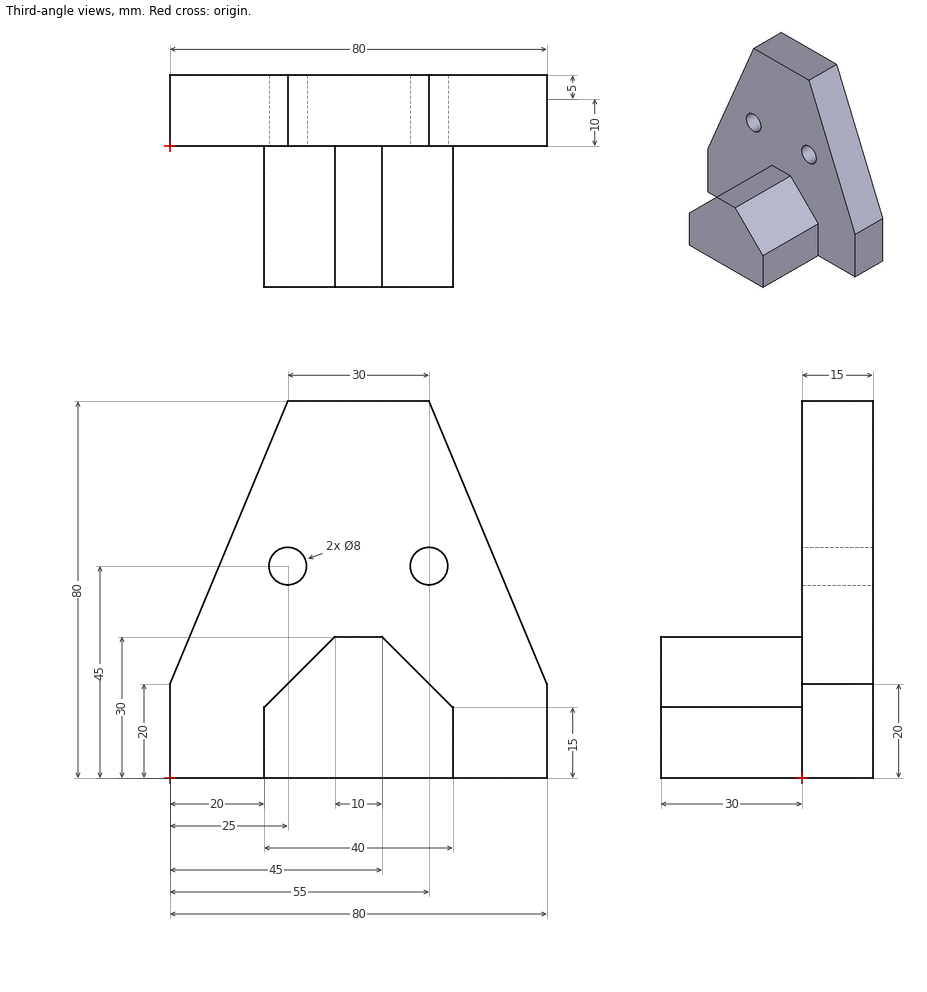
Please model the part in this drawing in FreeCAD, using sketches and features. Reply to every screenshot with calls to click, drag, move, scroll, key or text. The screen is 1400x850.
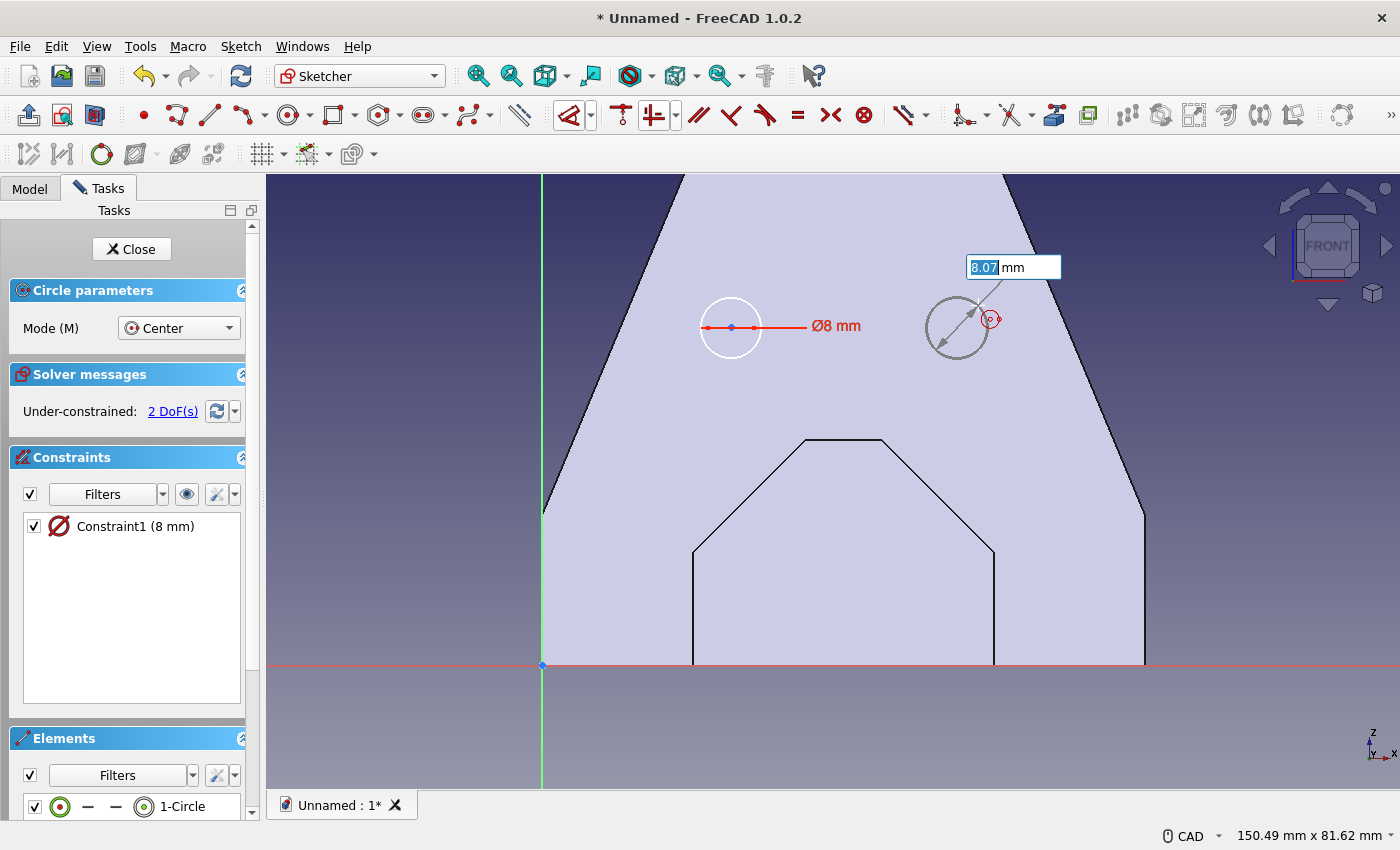
text(8)
key(Return)
key(Escape)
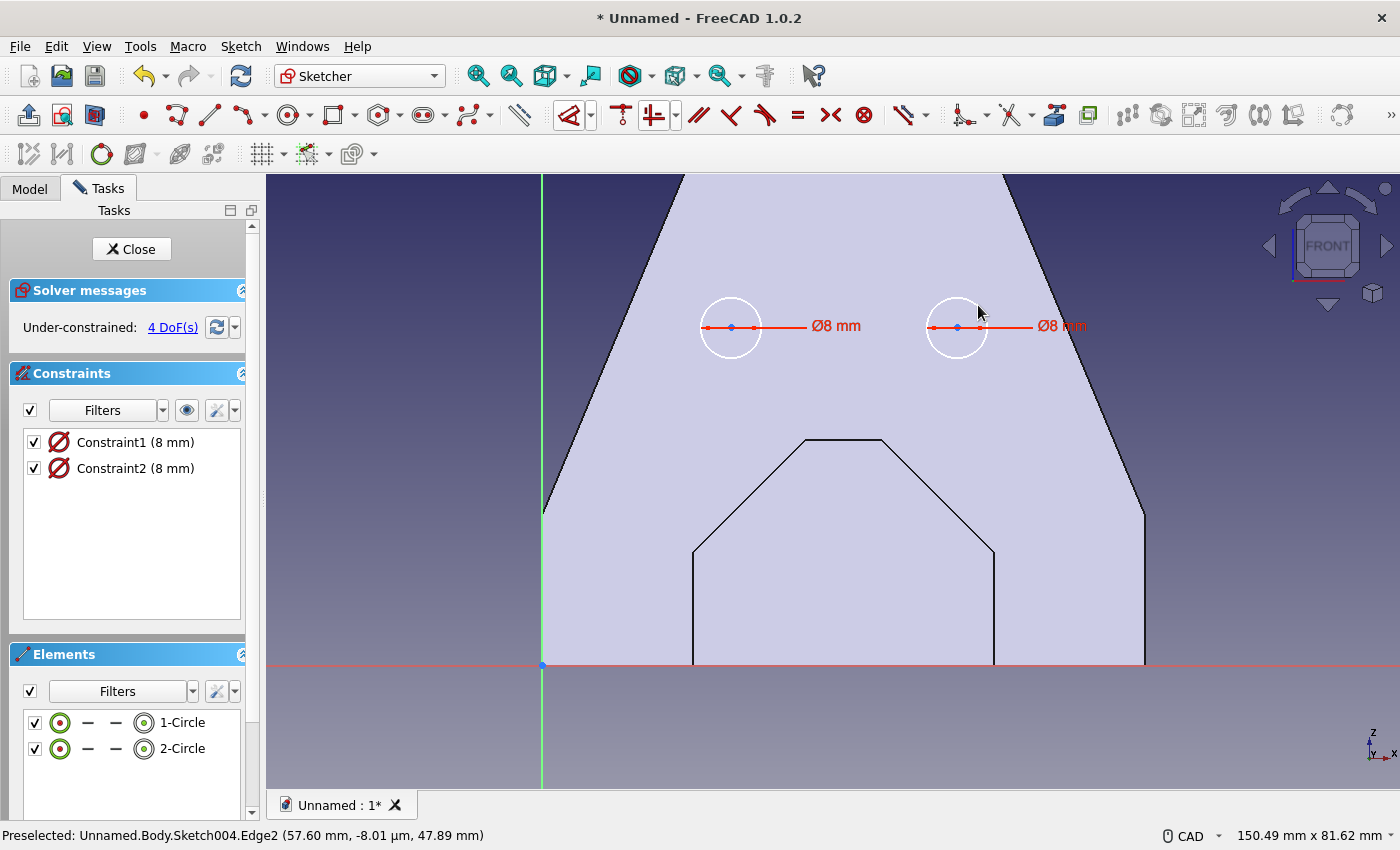
click(731, 328)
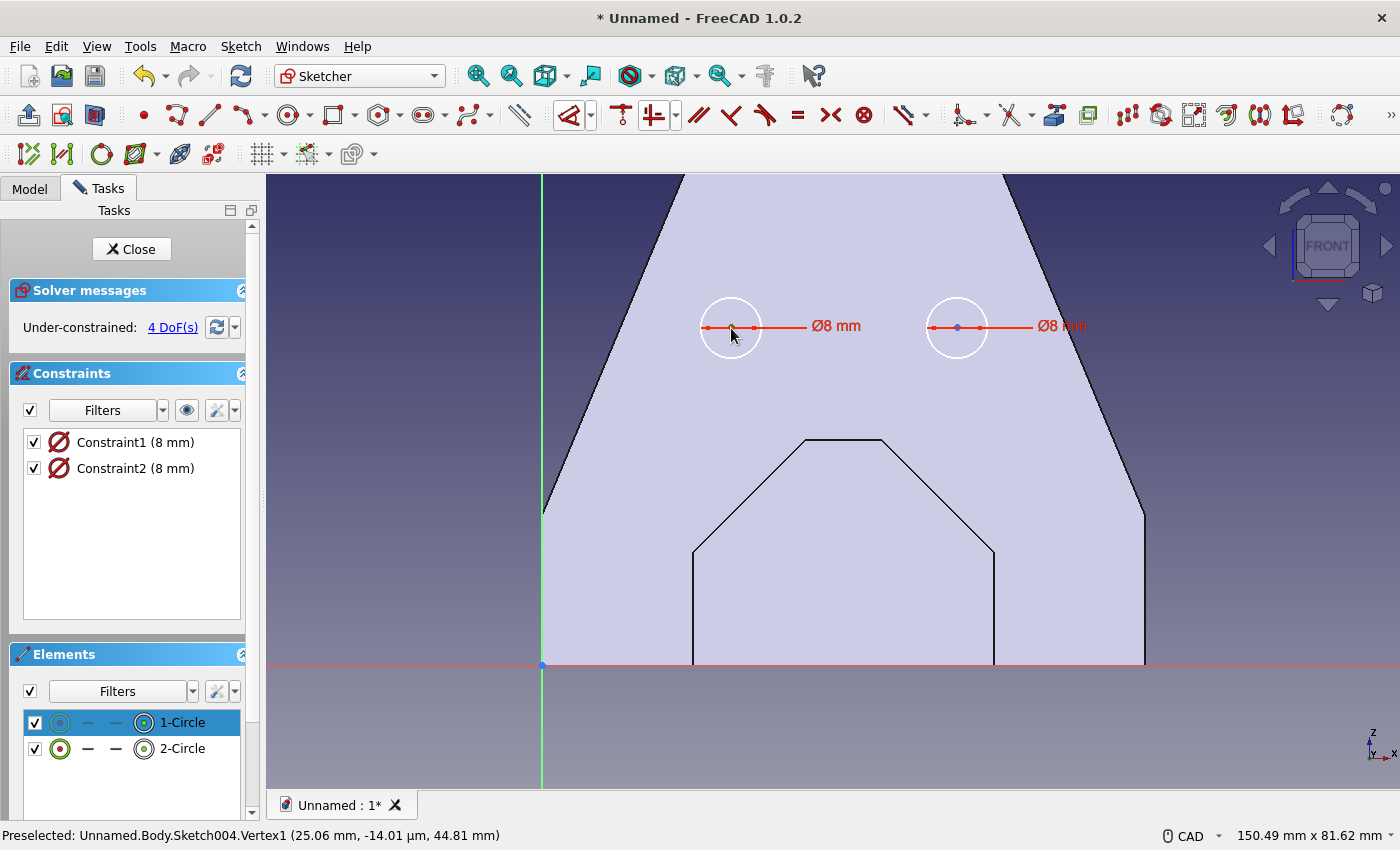
click(957, 328)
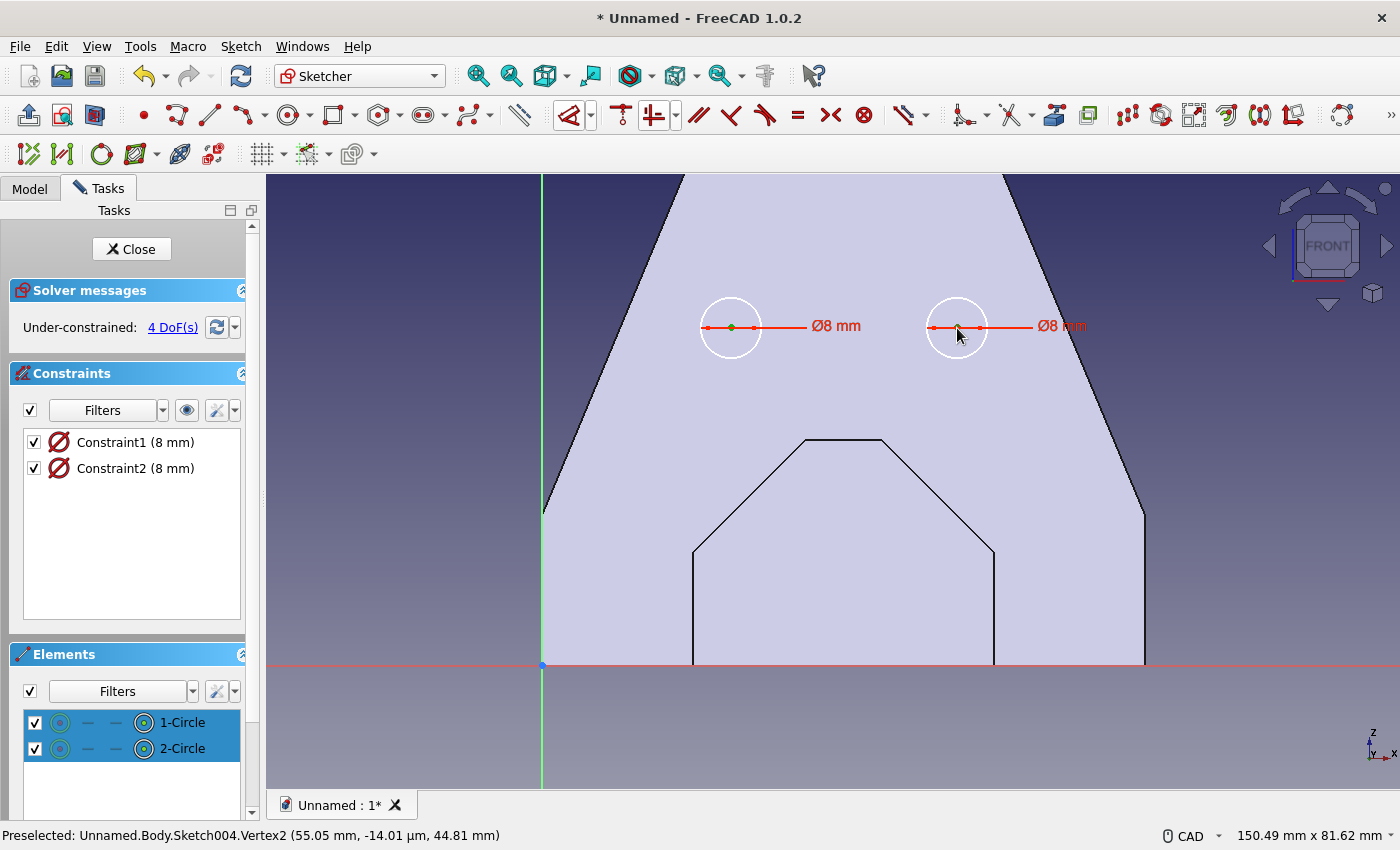
key(h)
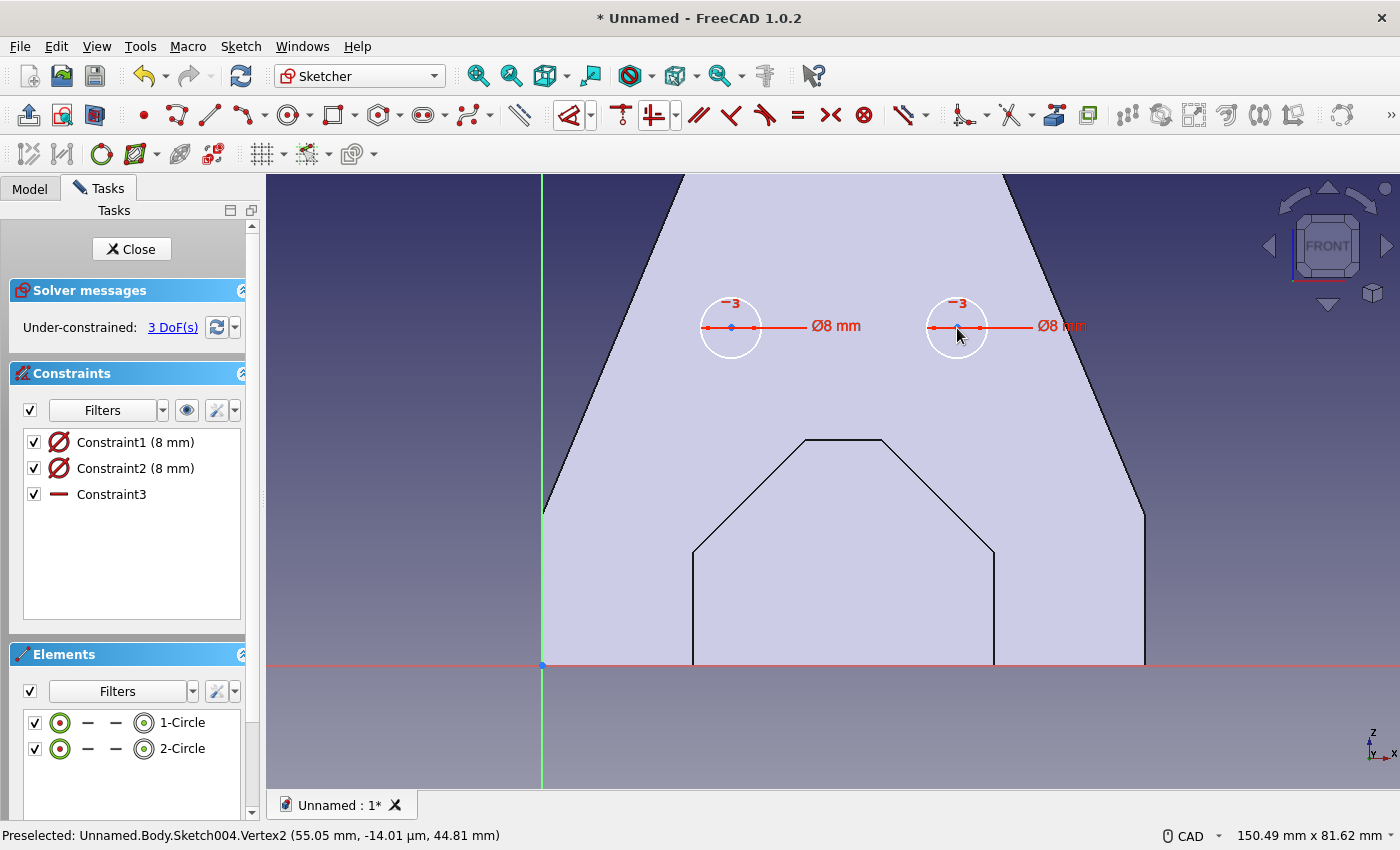
click(731, 328)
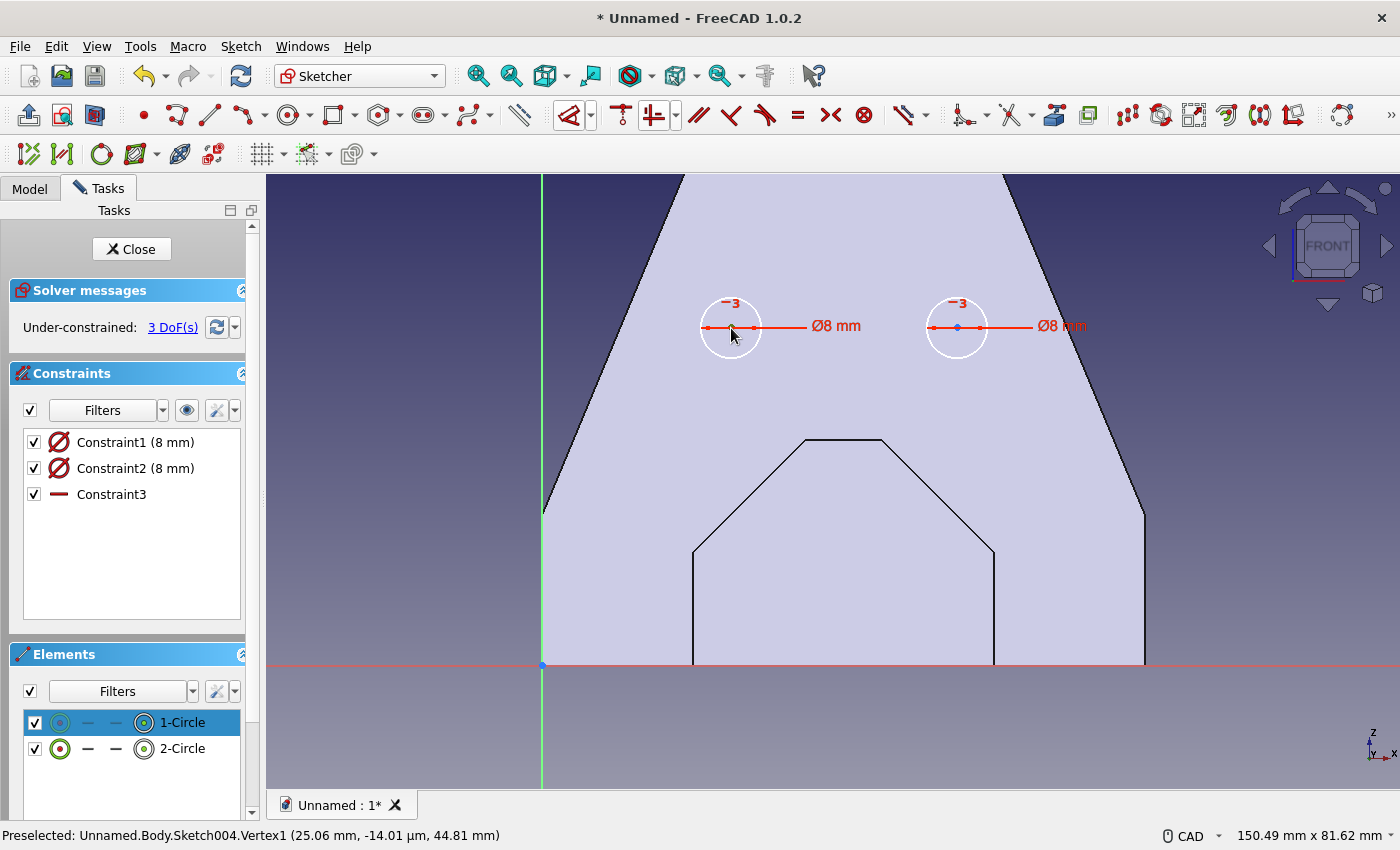
key(l)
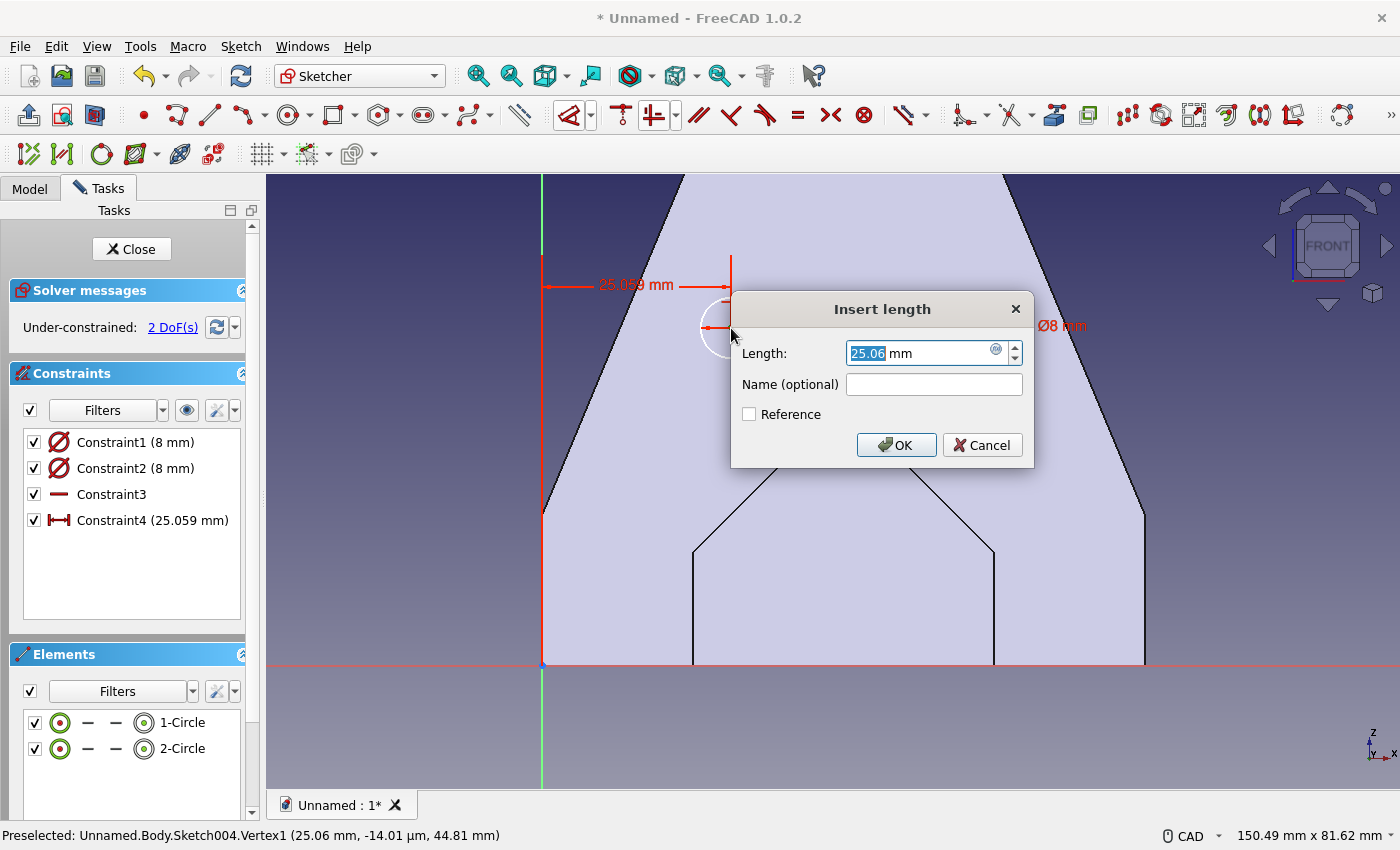
text(25)
key(Return)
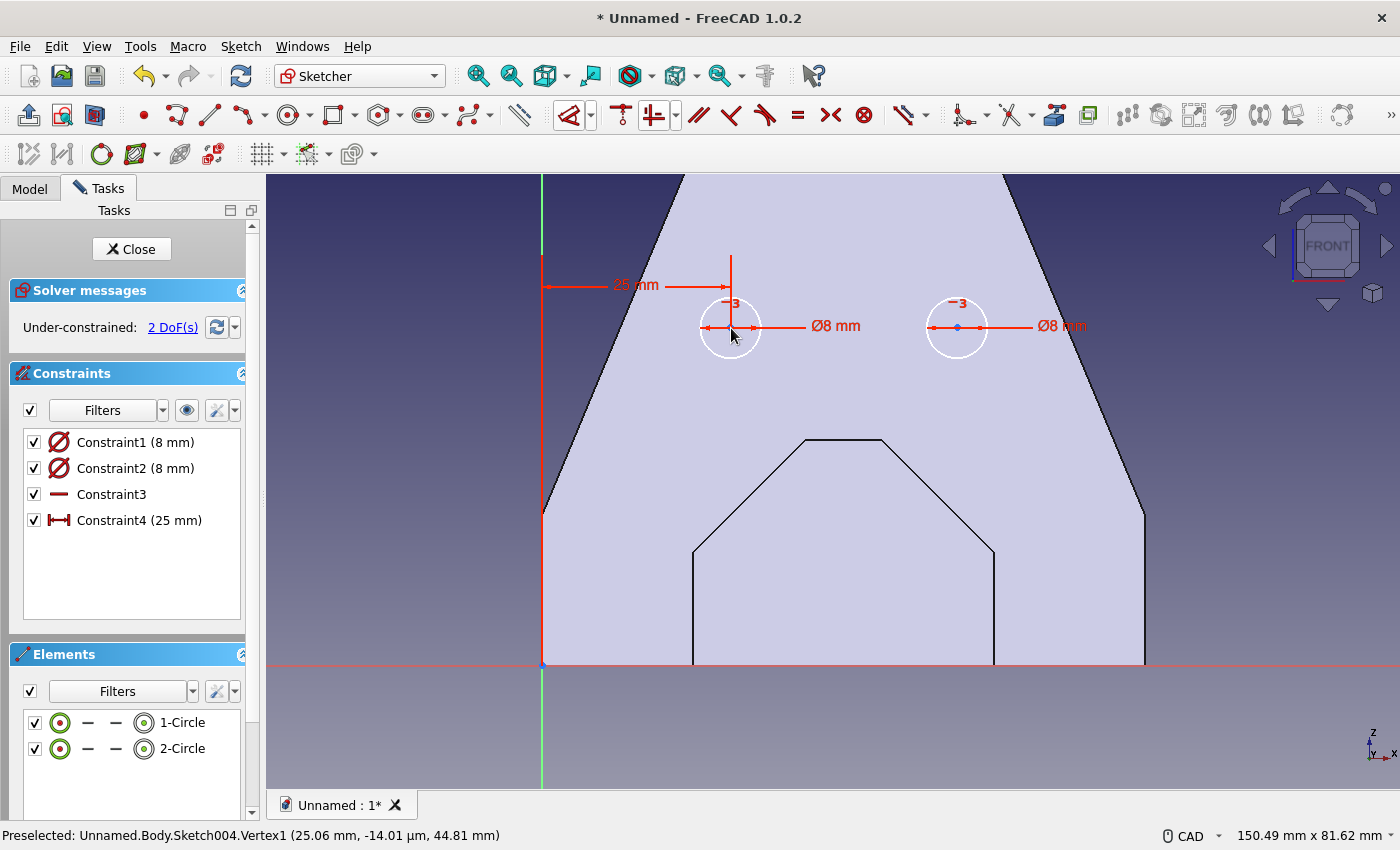
click(731, 328)